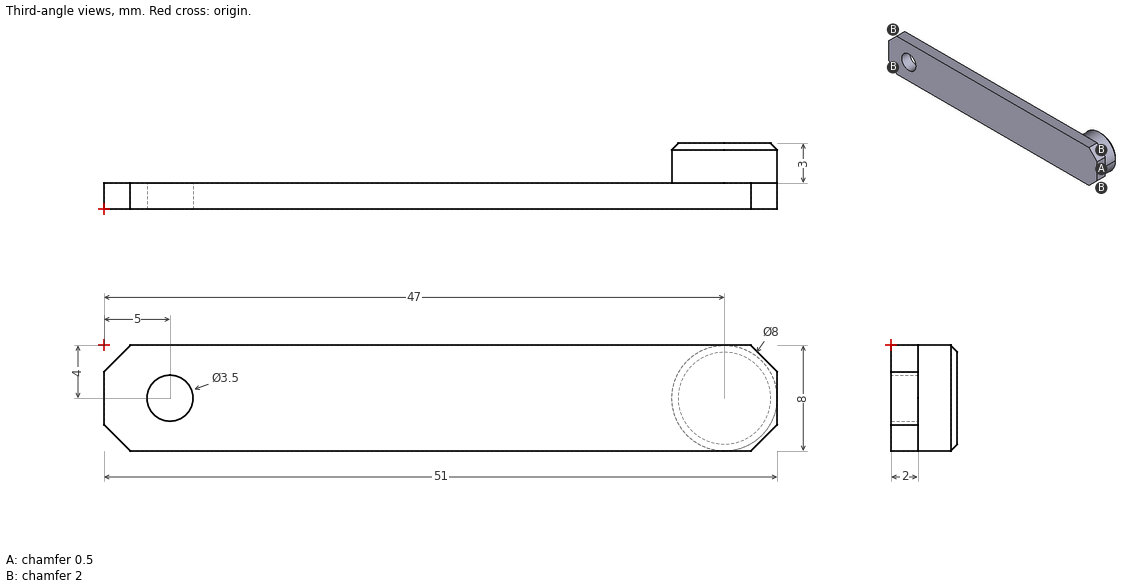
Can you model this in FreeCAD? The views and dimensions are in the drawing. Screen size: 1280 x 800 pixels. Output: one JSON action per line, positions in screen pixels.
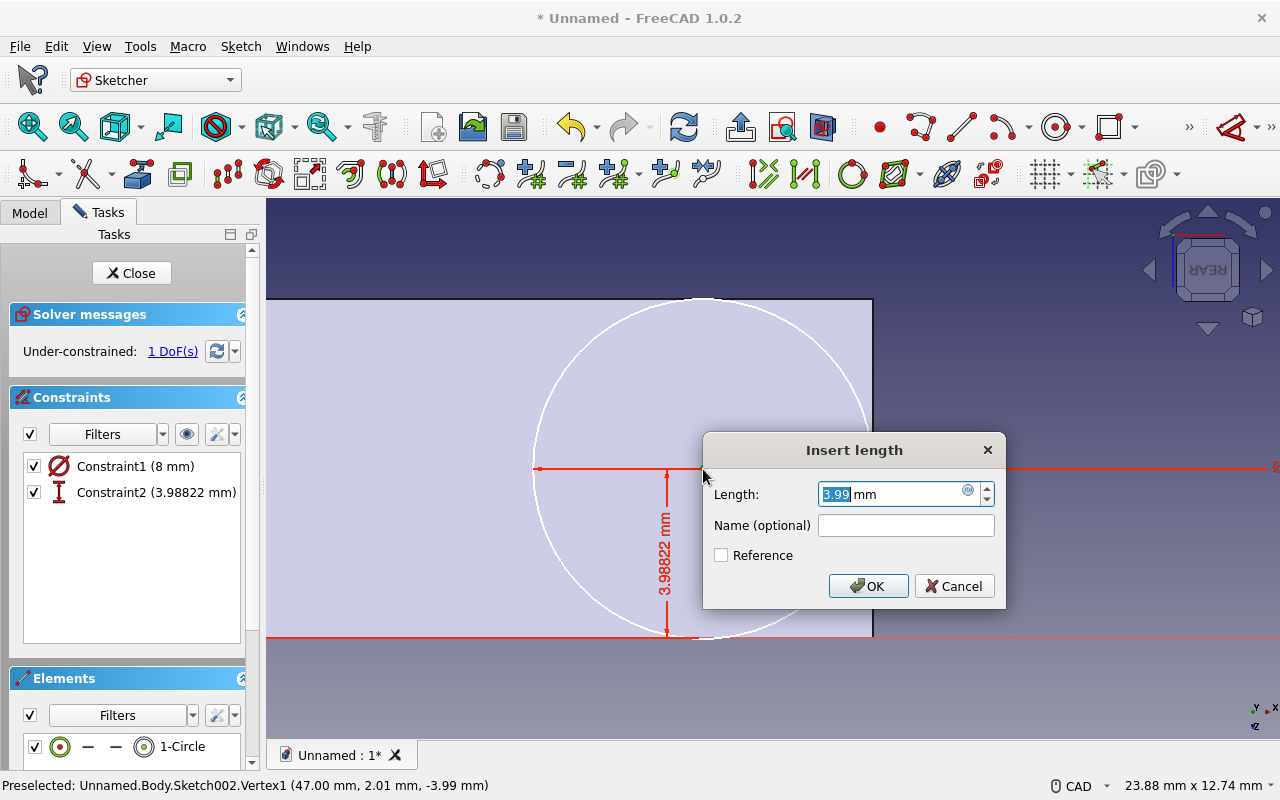
{"action": "type", "text": "4"}
{"action": "key", "text": "Return"}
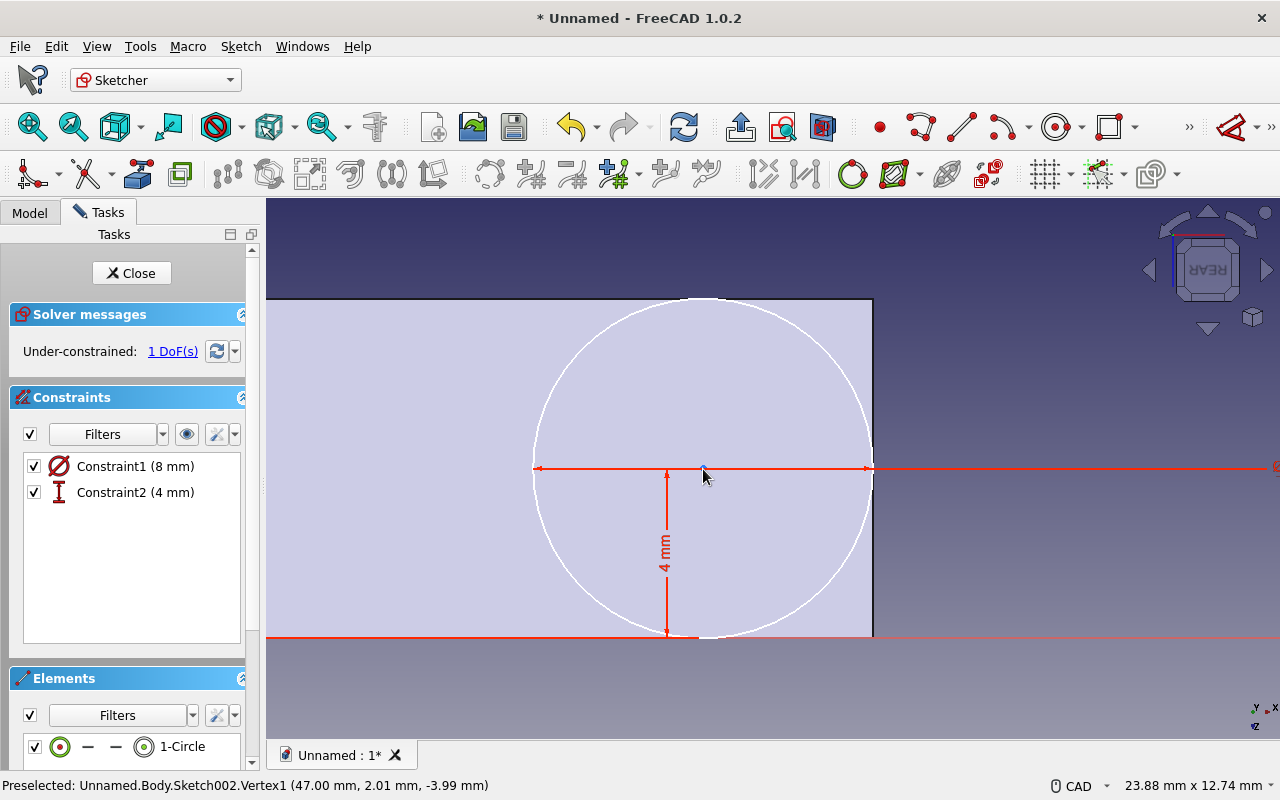
{"action": "left_click", "coordinate": [703, 468]}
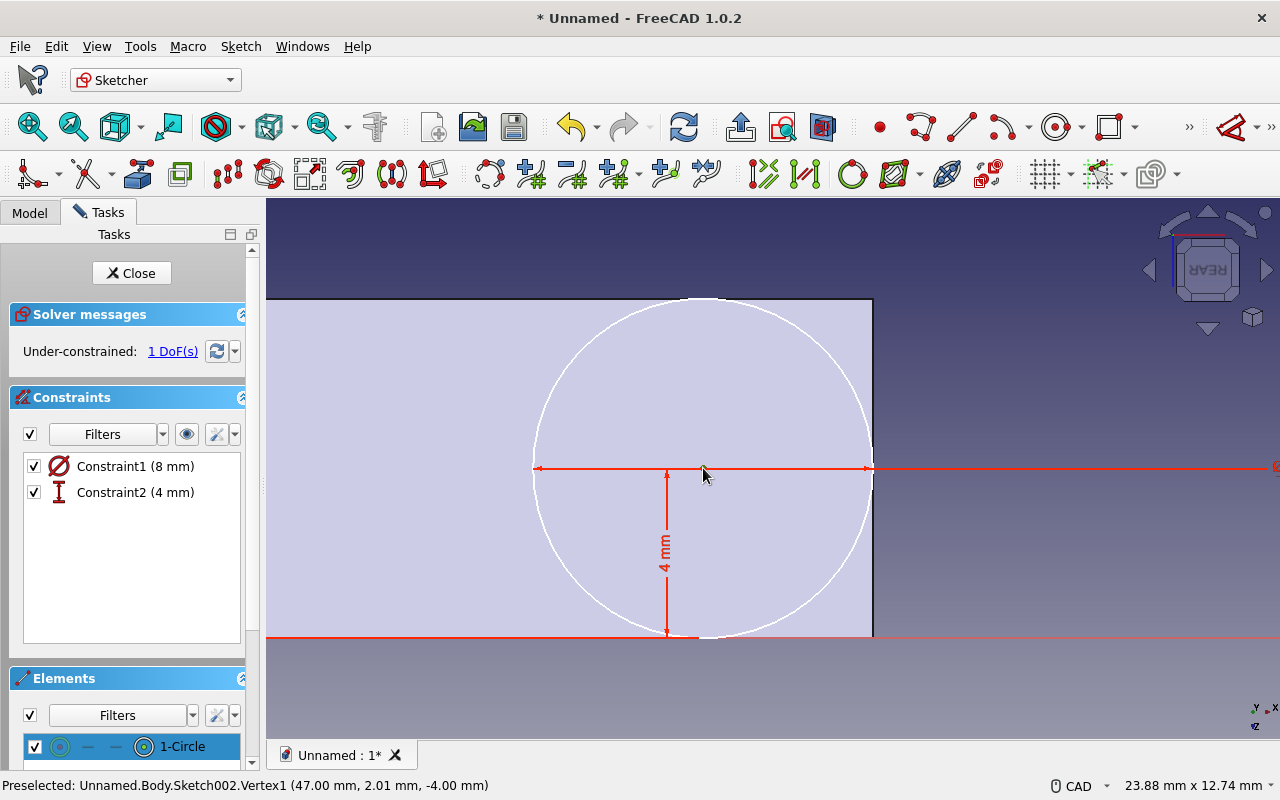
{"action": "key", "text": "l"}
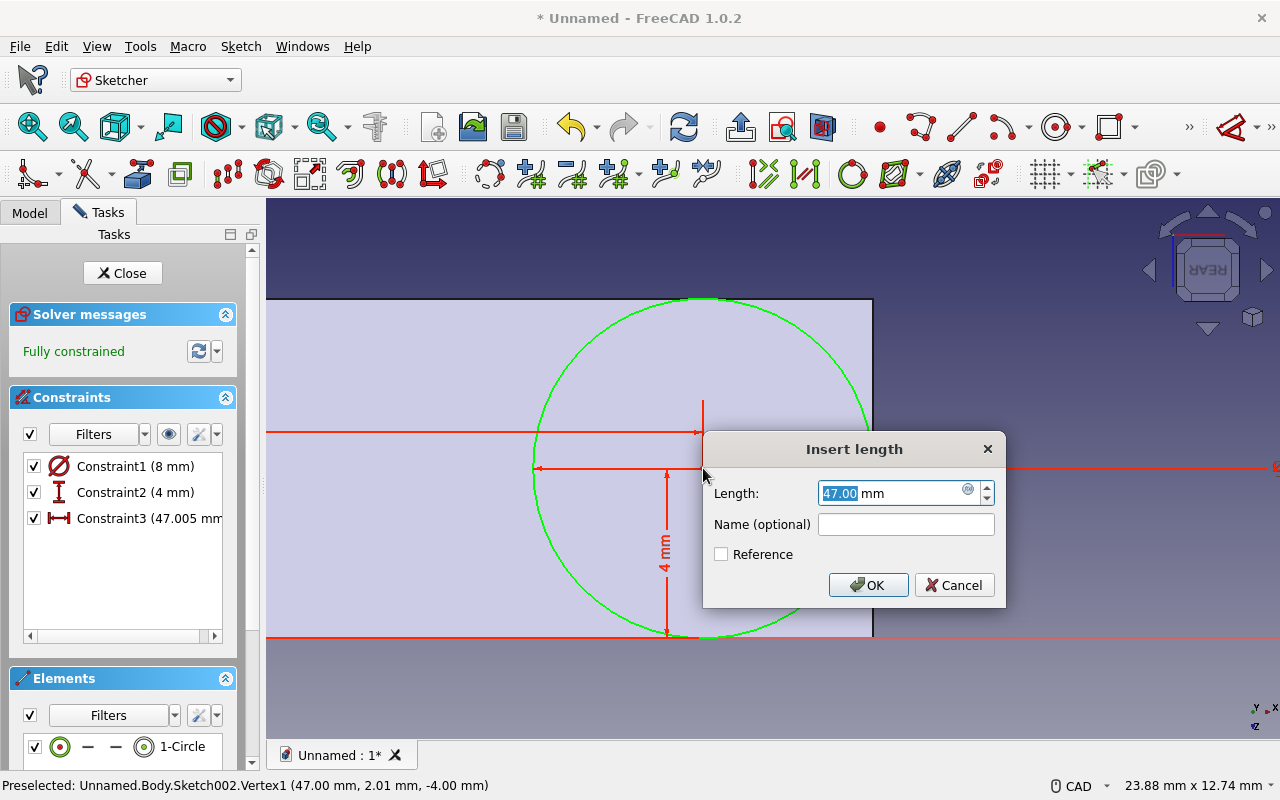
{"action": "type", "text": "47"}
{"action": "key", "text": "Return"}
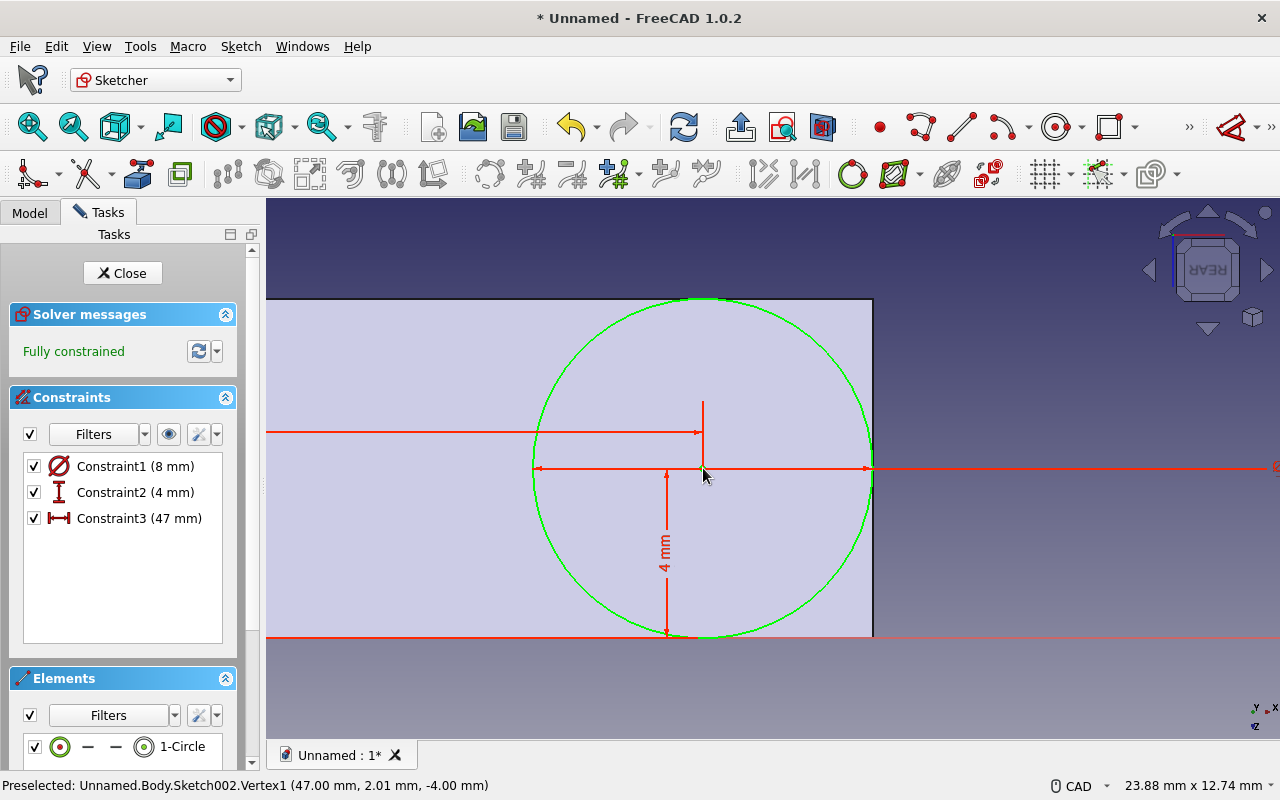
{"action": "left_click", "coordinate": [123, 273]}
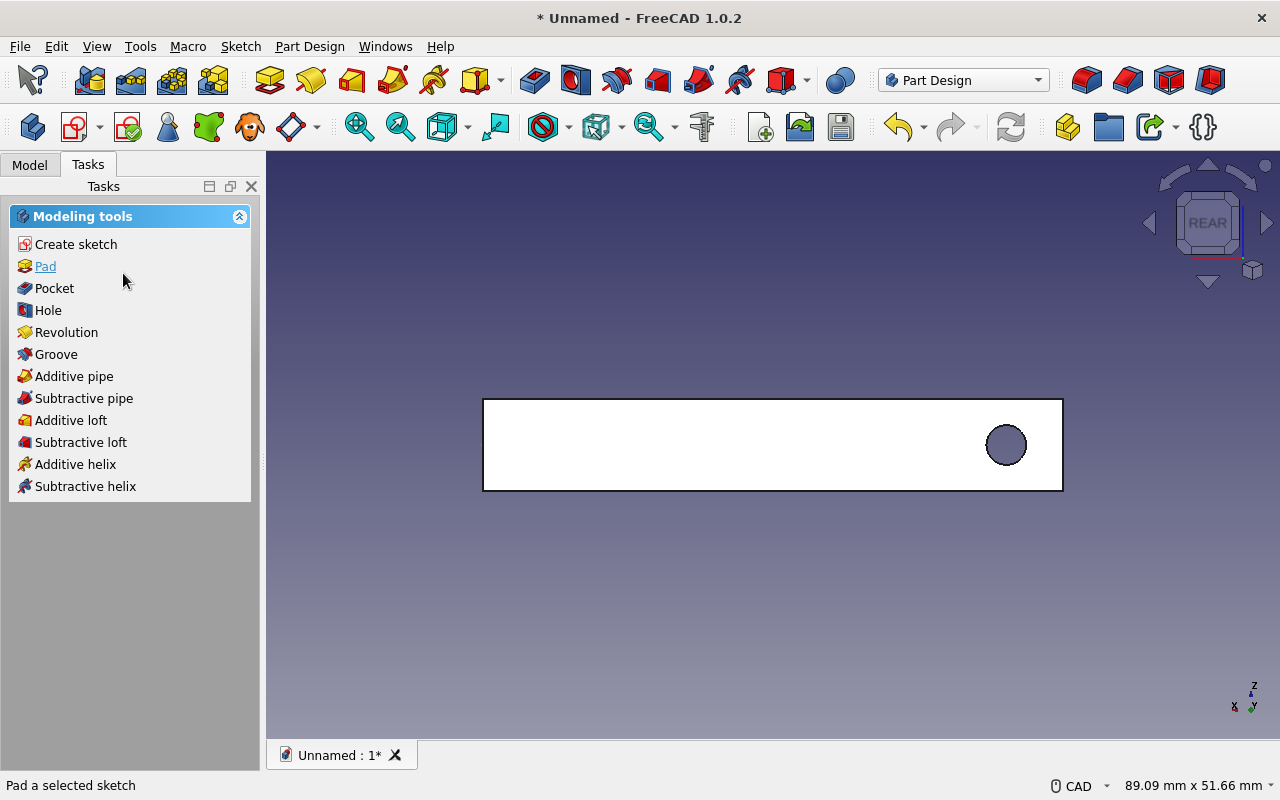
{"action": "left_click", "coordinate": [270, 80]}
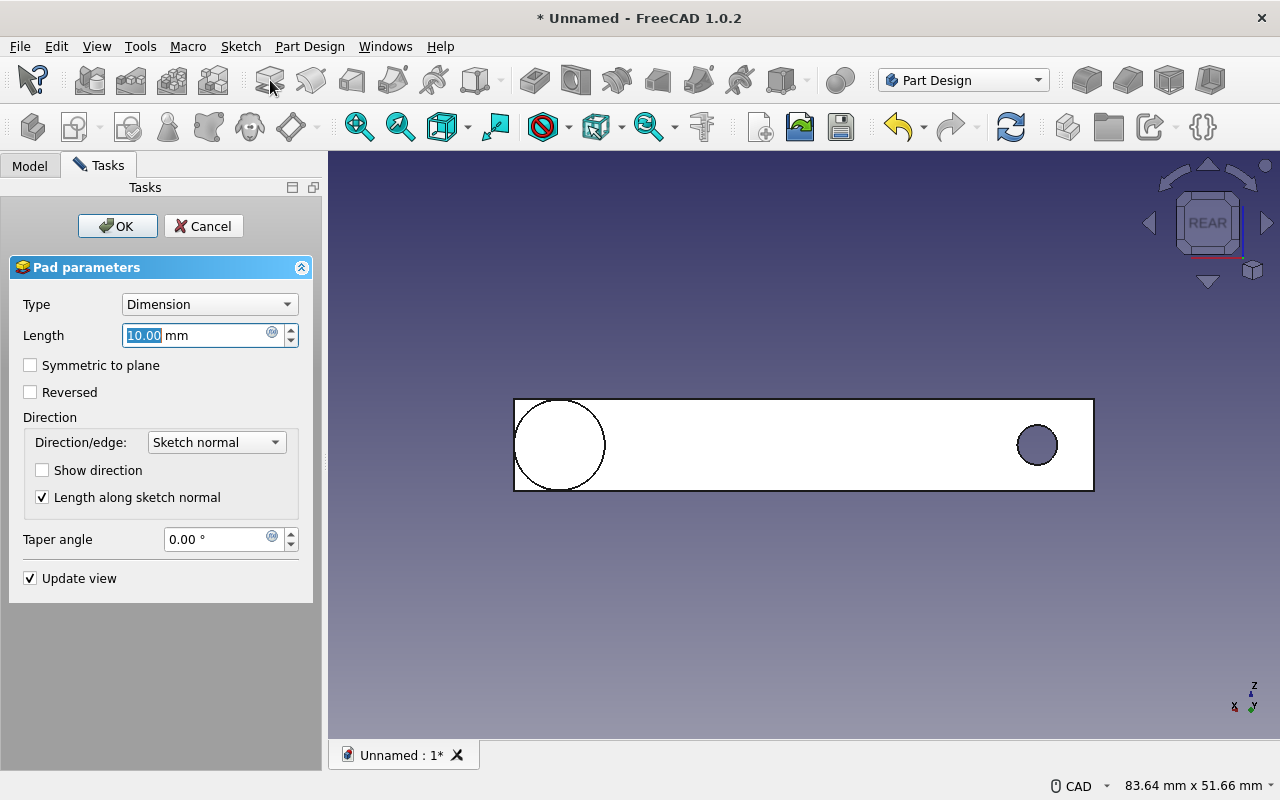
{"action": "type", "text": "3"}
{"action": "key", "text": "Tab"}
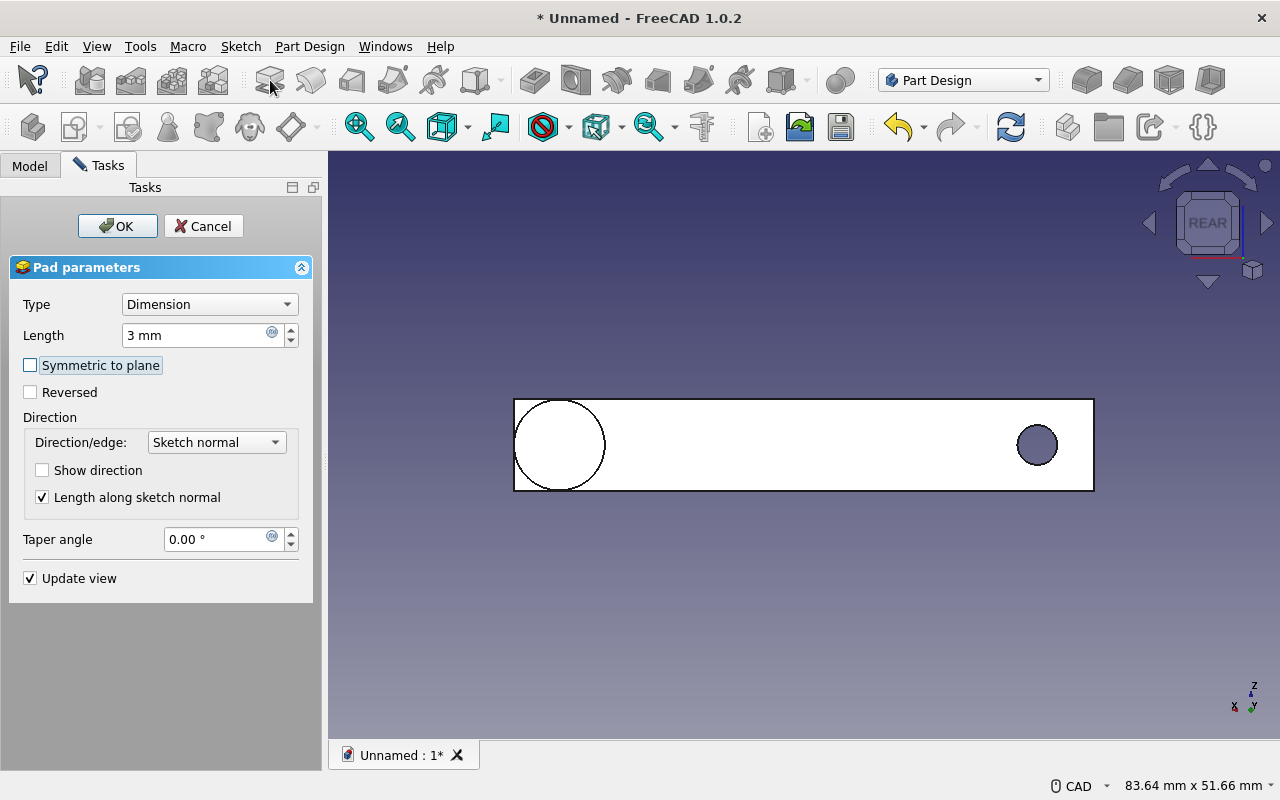
{"action": "left_click", "coordinate": [118, 226]}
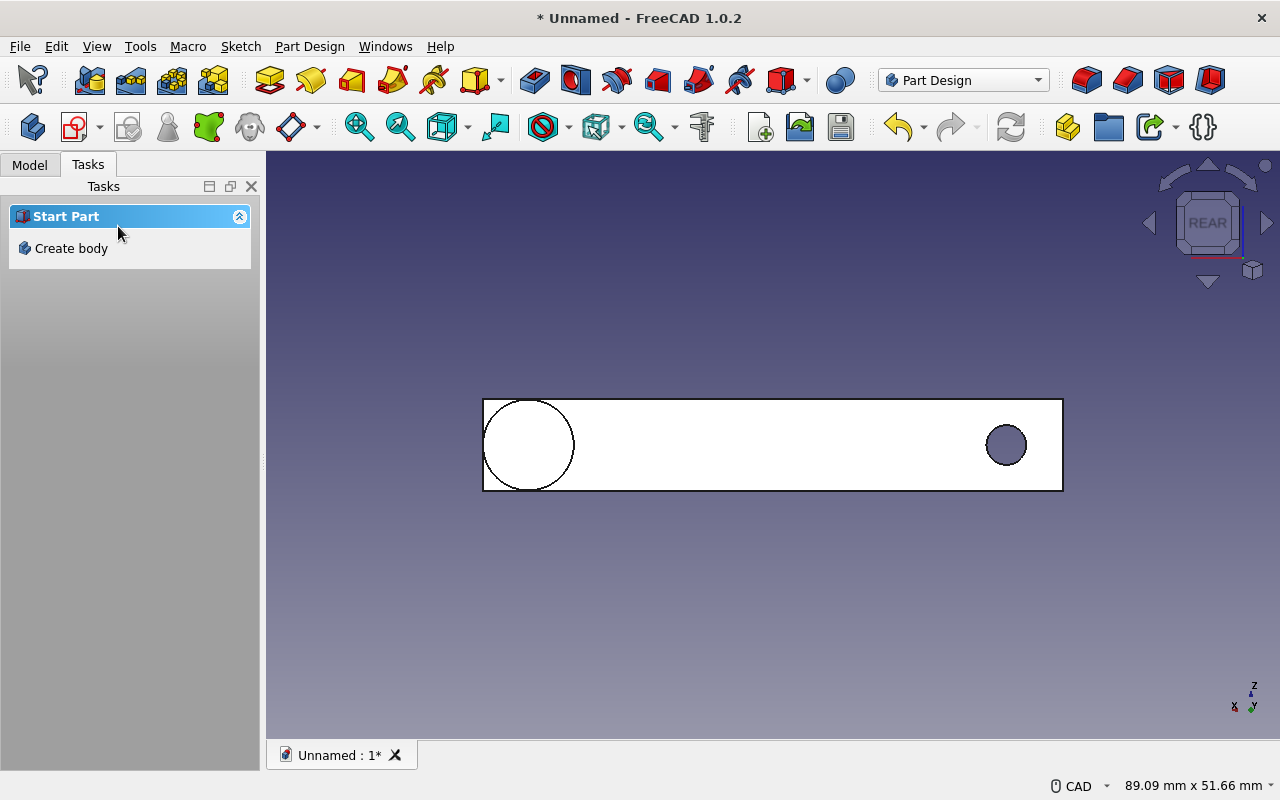
{"action": "left_click", "coordinate": [574, 444]}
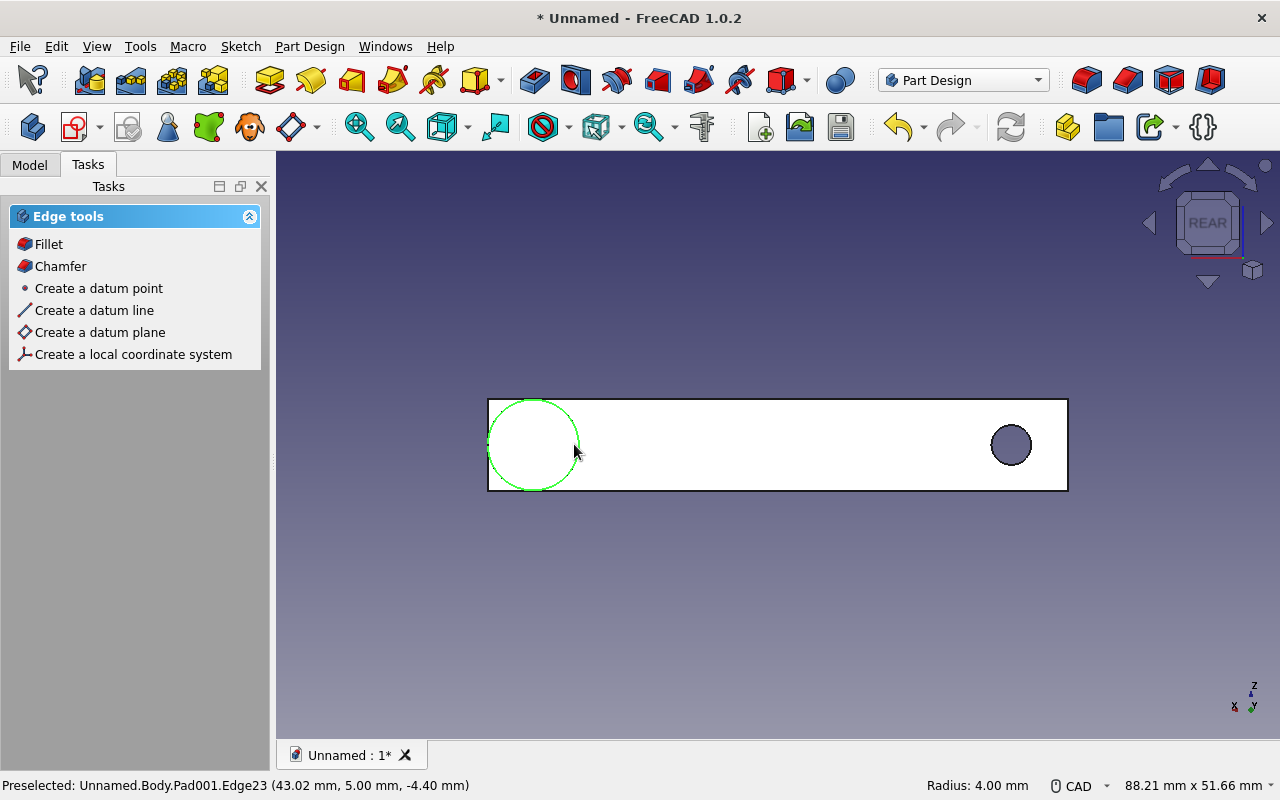
{"action": "left_click", "coordinate": [1128, 80]}